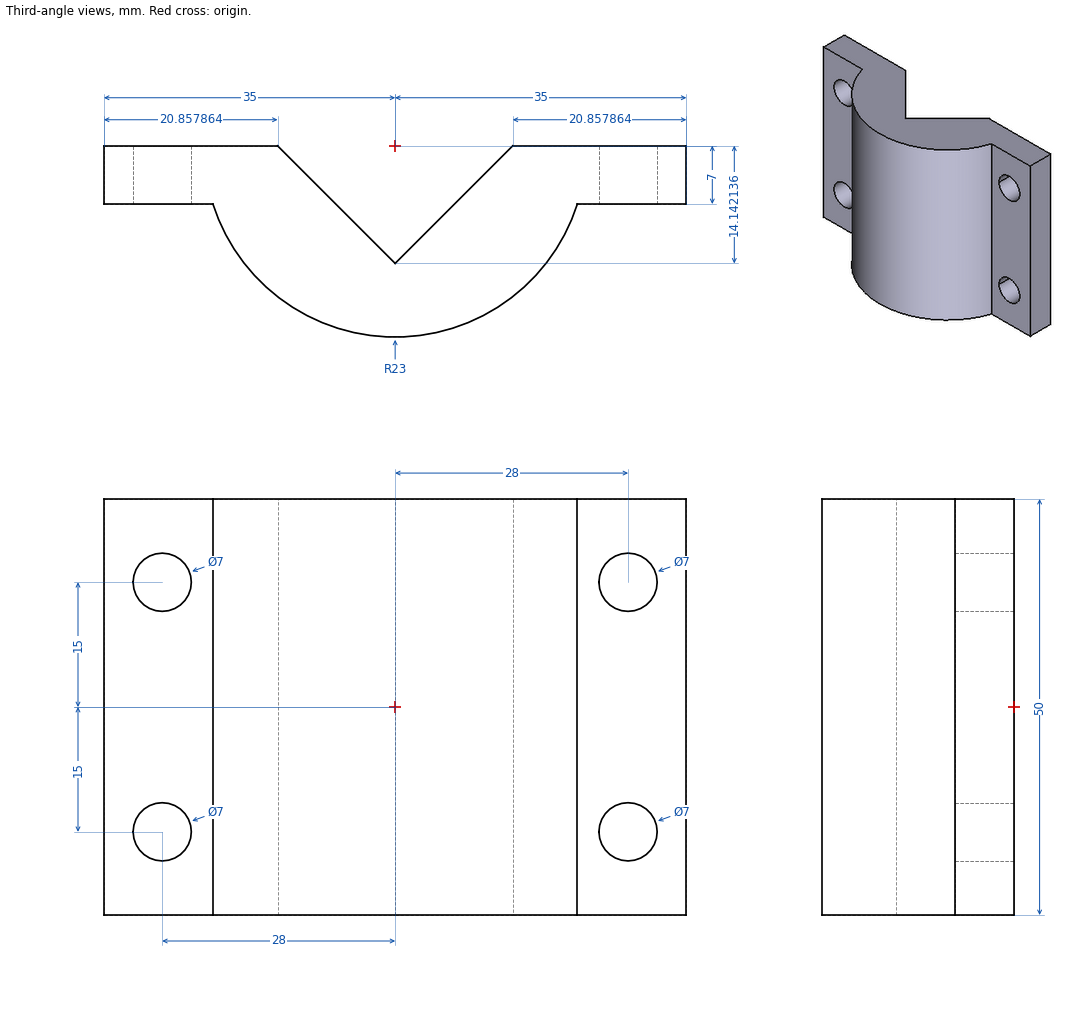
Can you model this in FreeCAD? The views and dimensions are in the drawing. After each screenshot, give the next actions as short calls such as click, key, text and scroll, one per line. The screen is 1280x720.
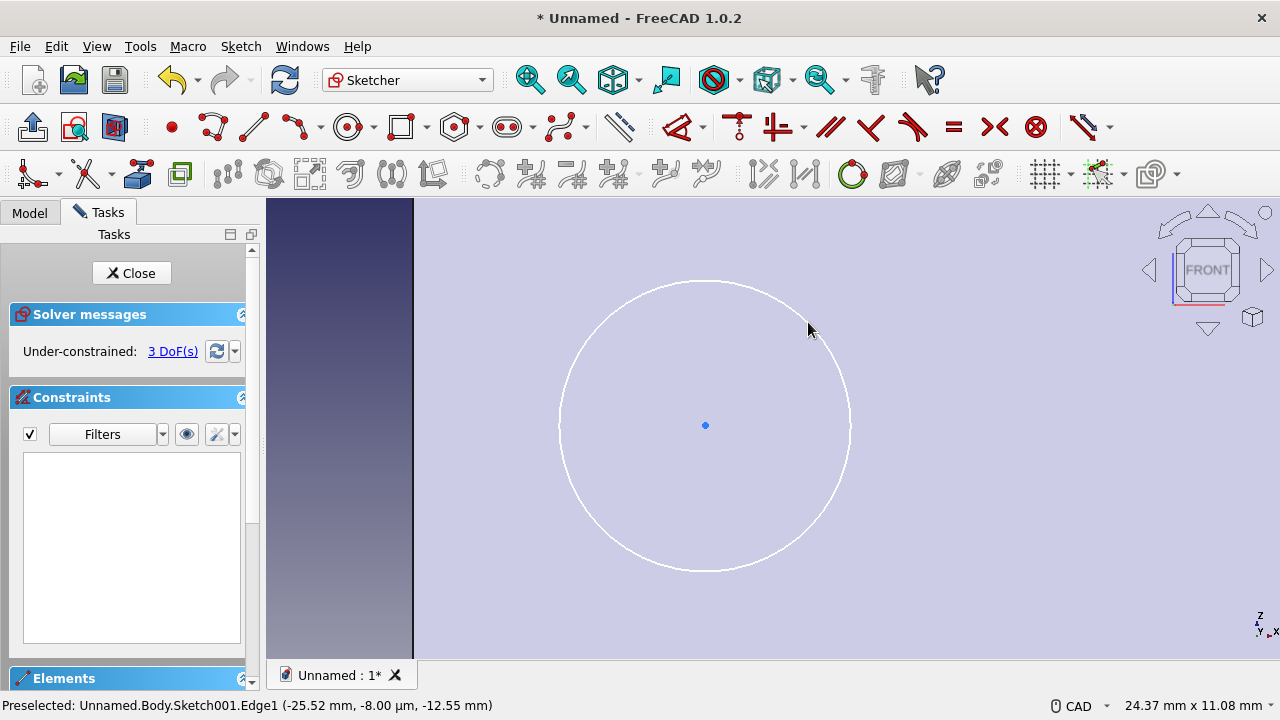
key(d)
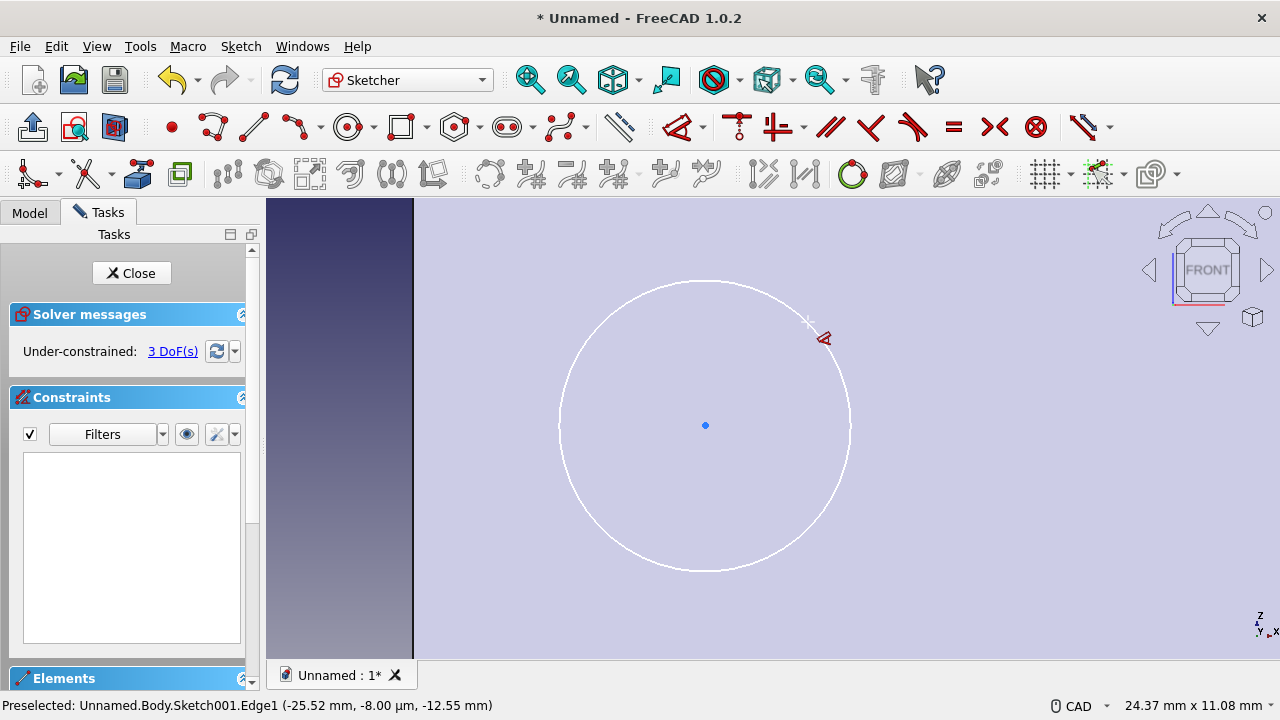
click(808, 323)
click(831, 300)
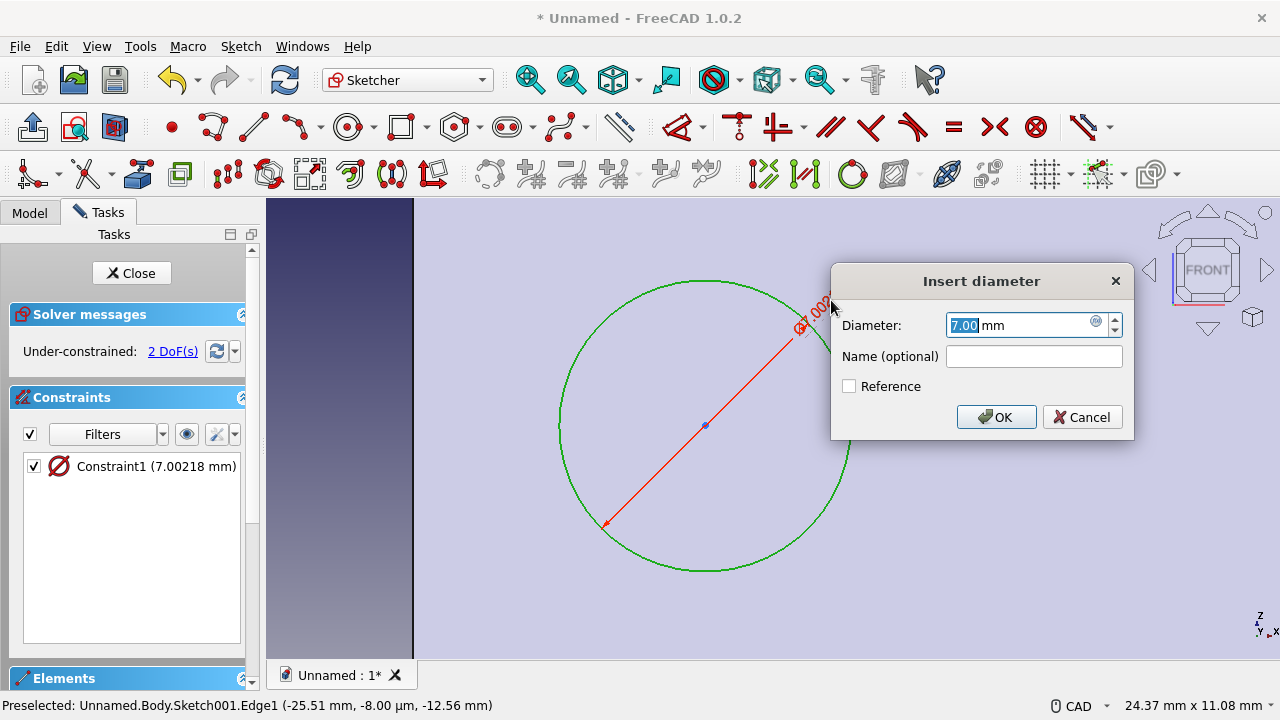
text(7)
key(Return)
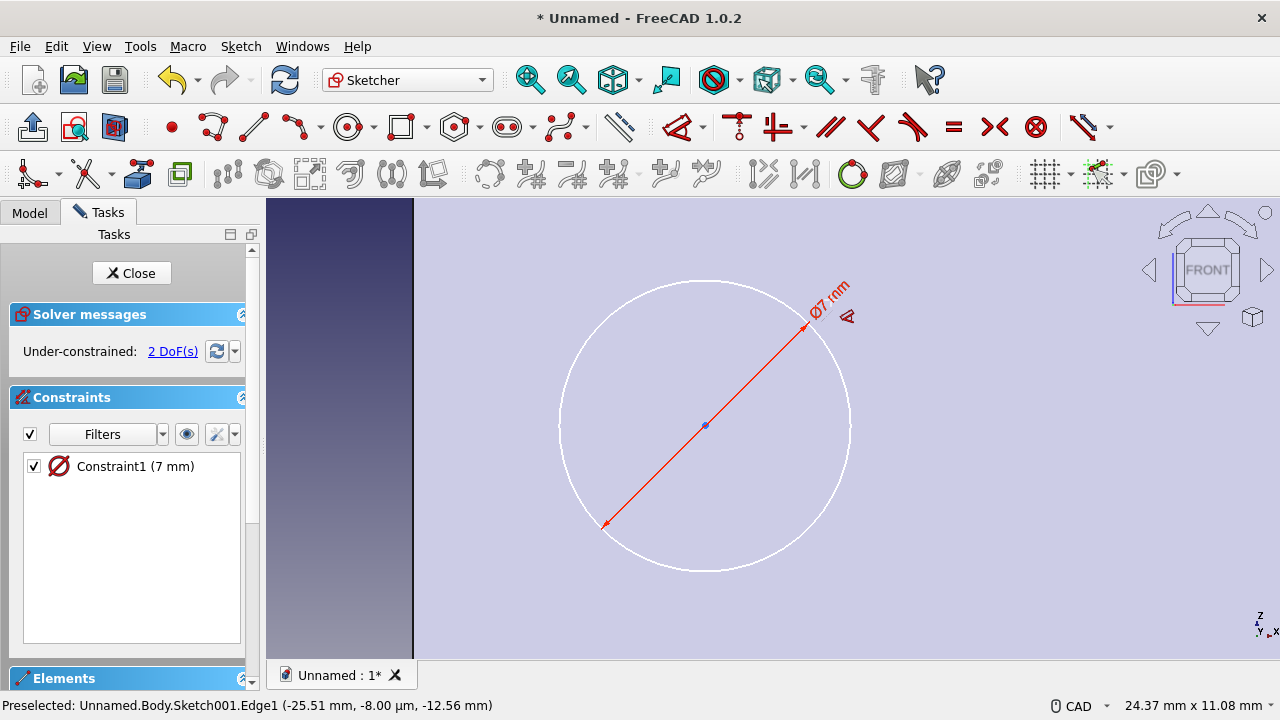
click(705, 426)
click(910, 460)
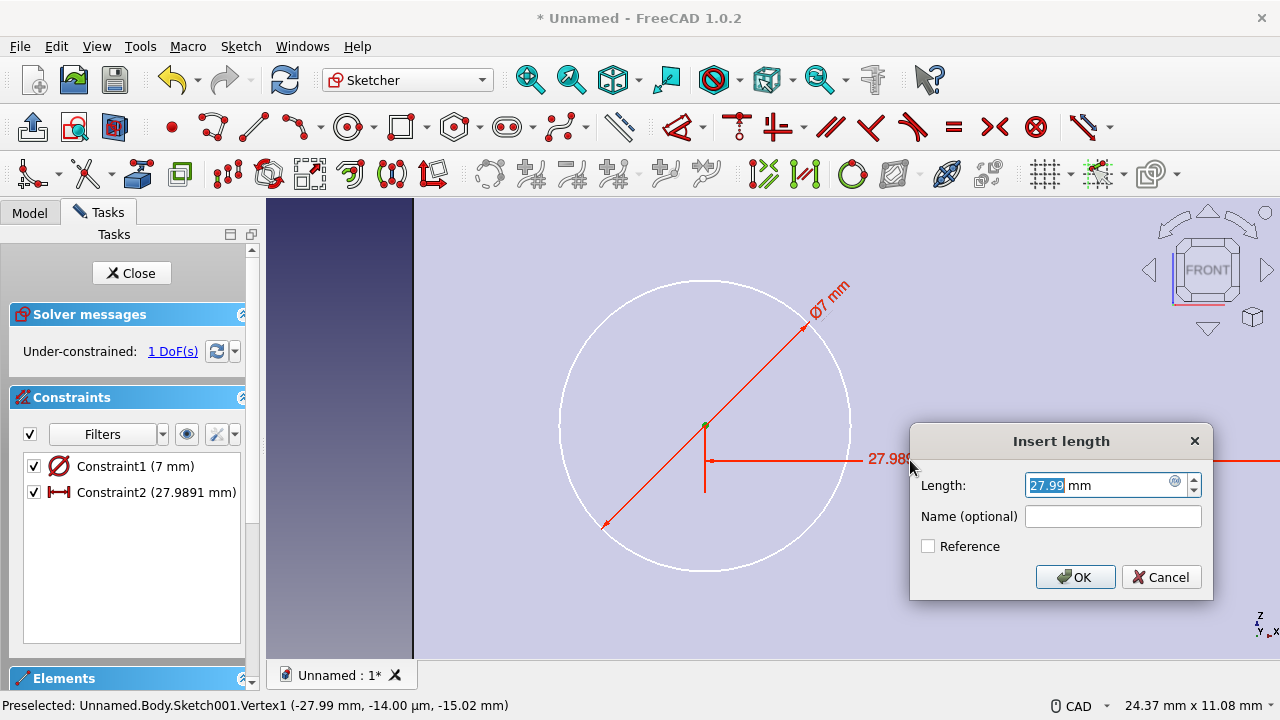
text(28)
key(Return)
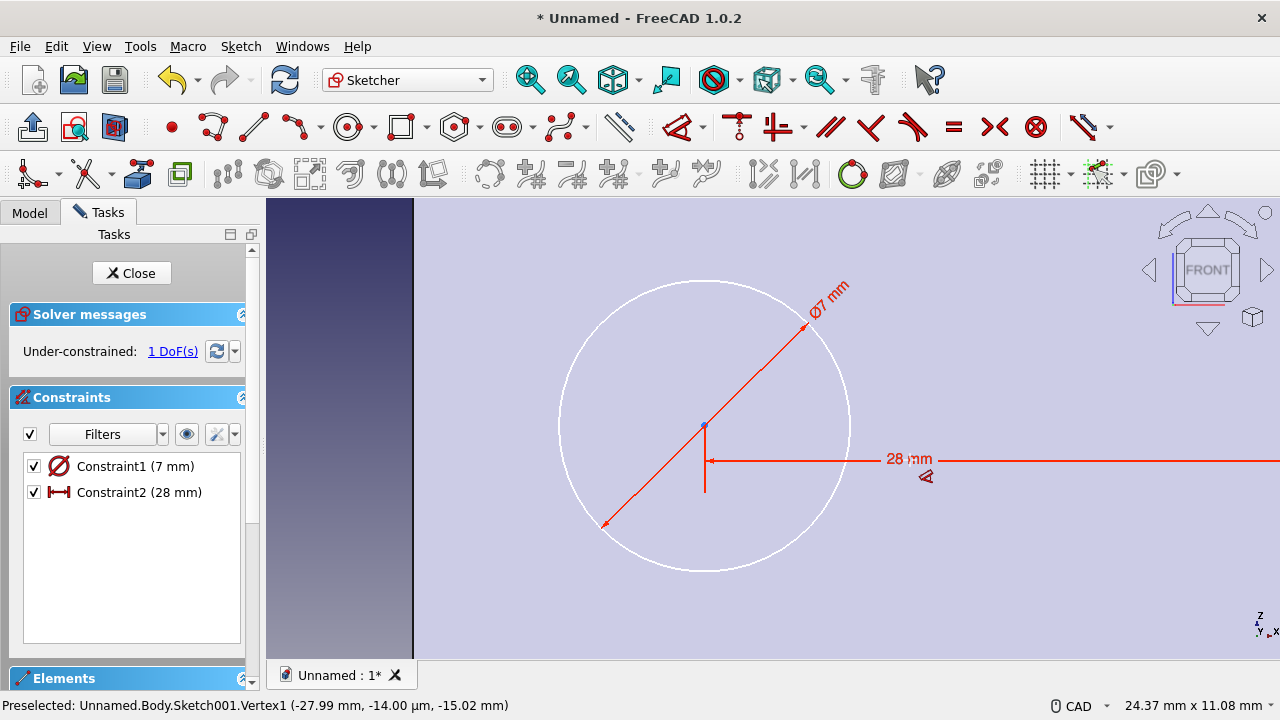
click(705, 426)
click(671, 326)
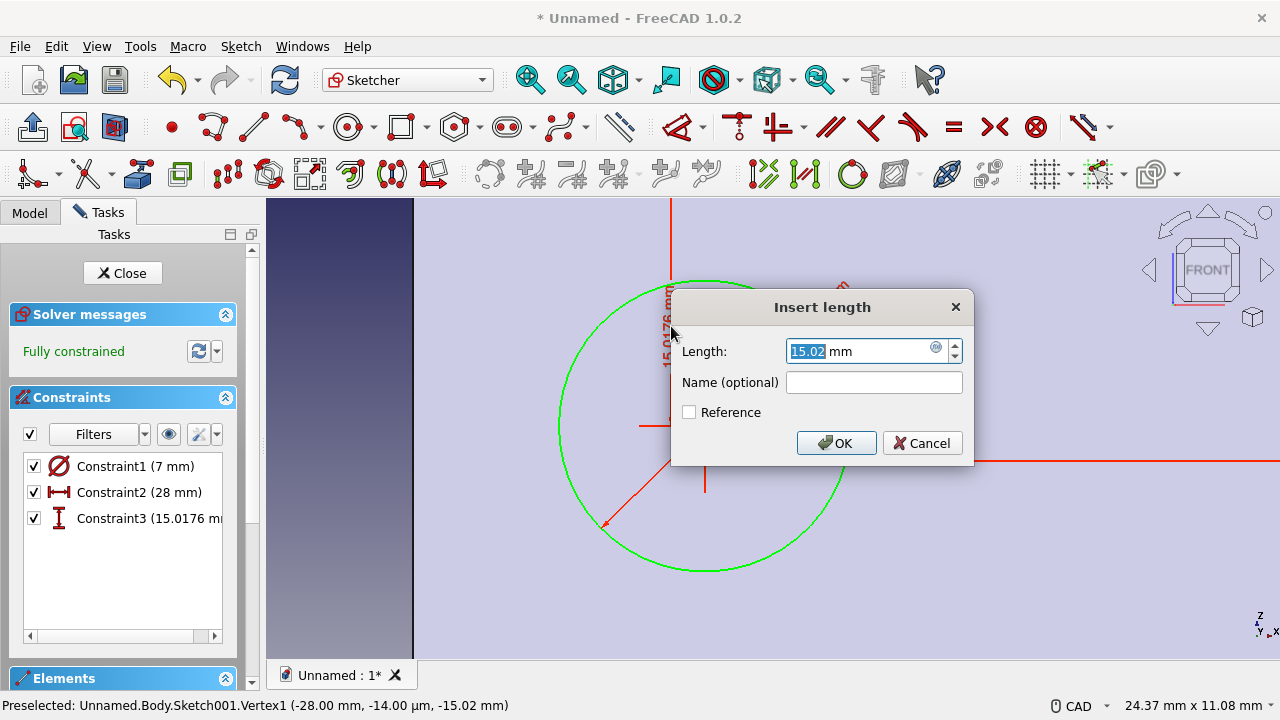
text(15)
key(Return)
key(Escape)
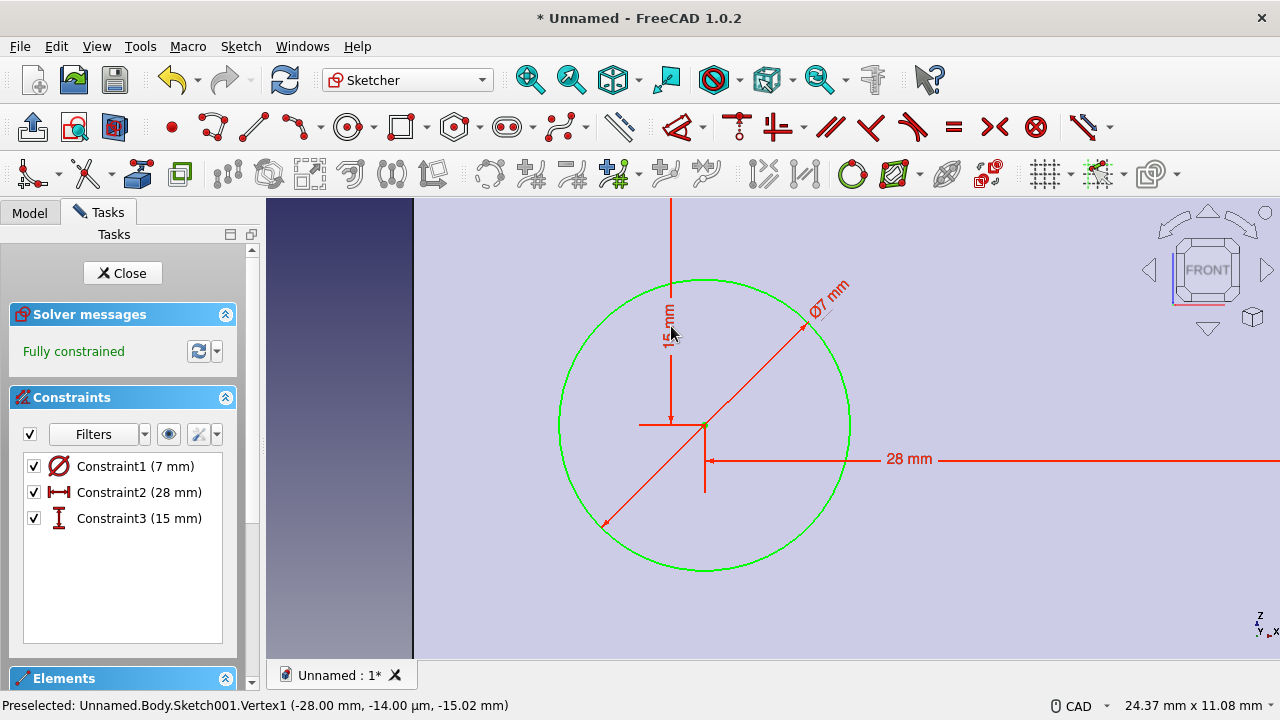
click(123, 273)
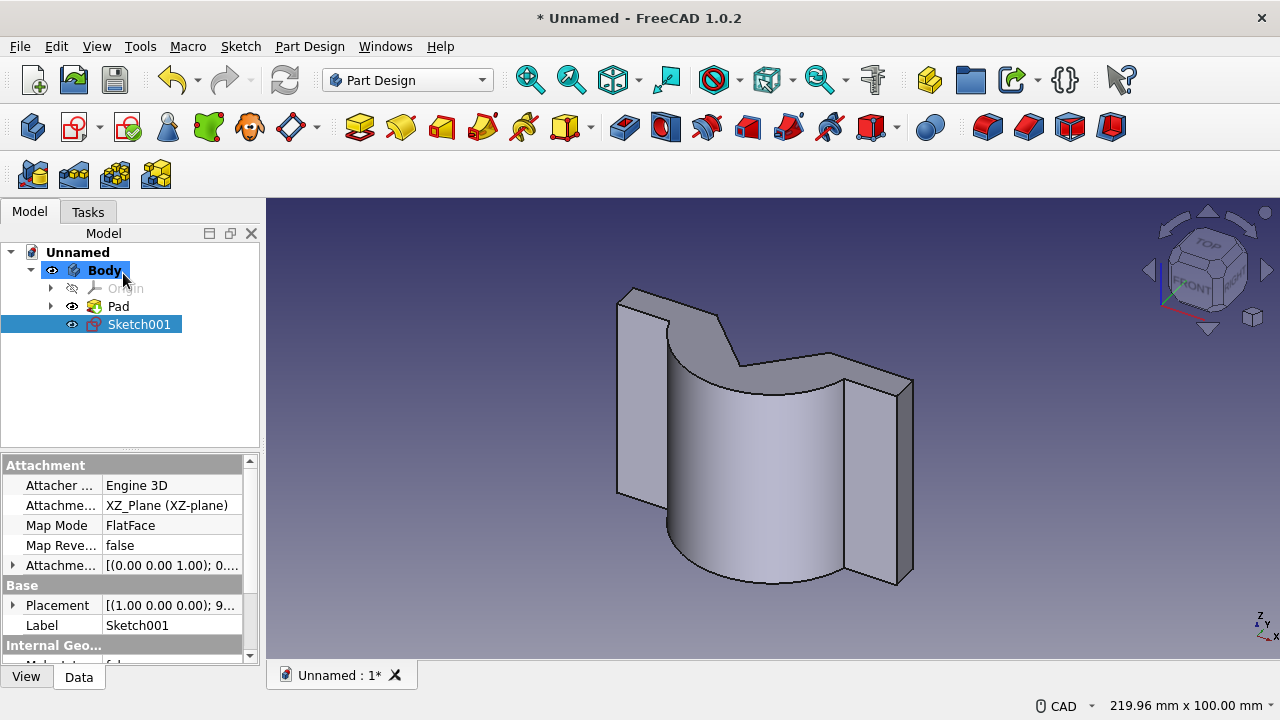
click(625, 128)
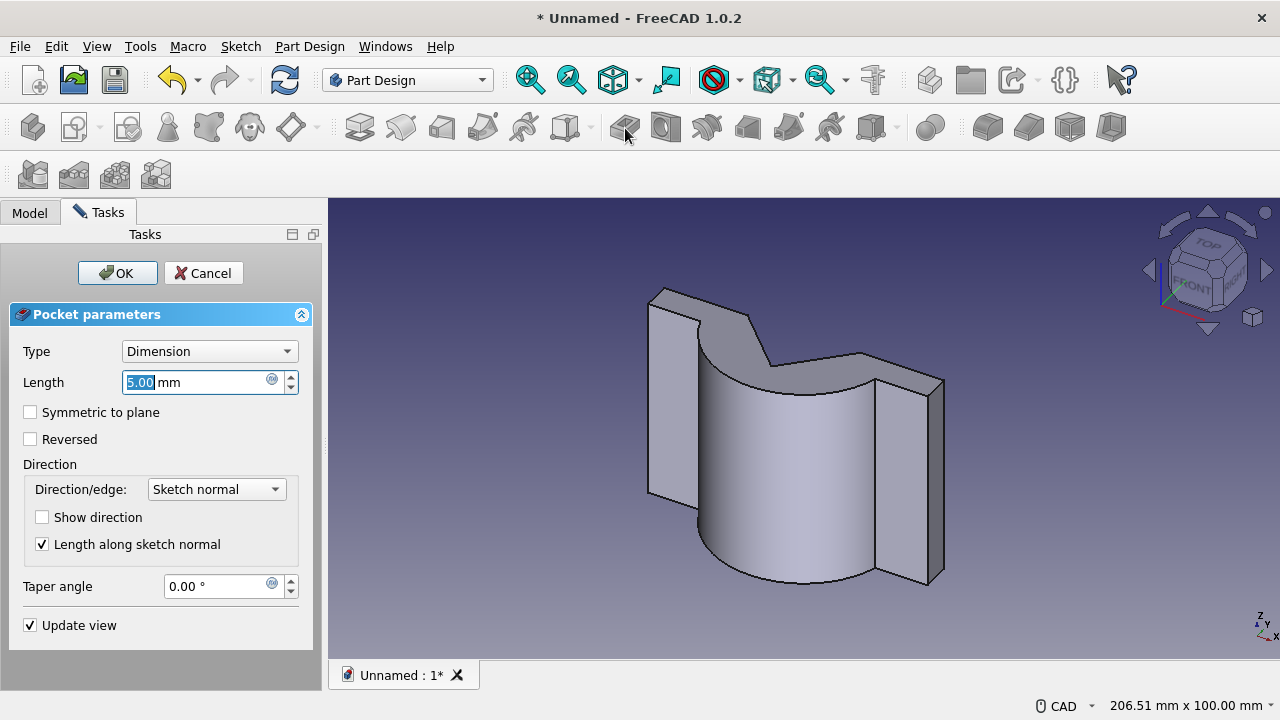
click(210, 352)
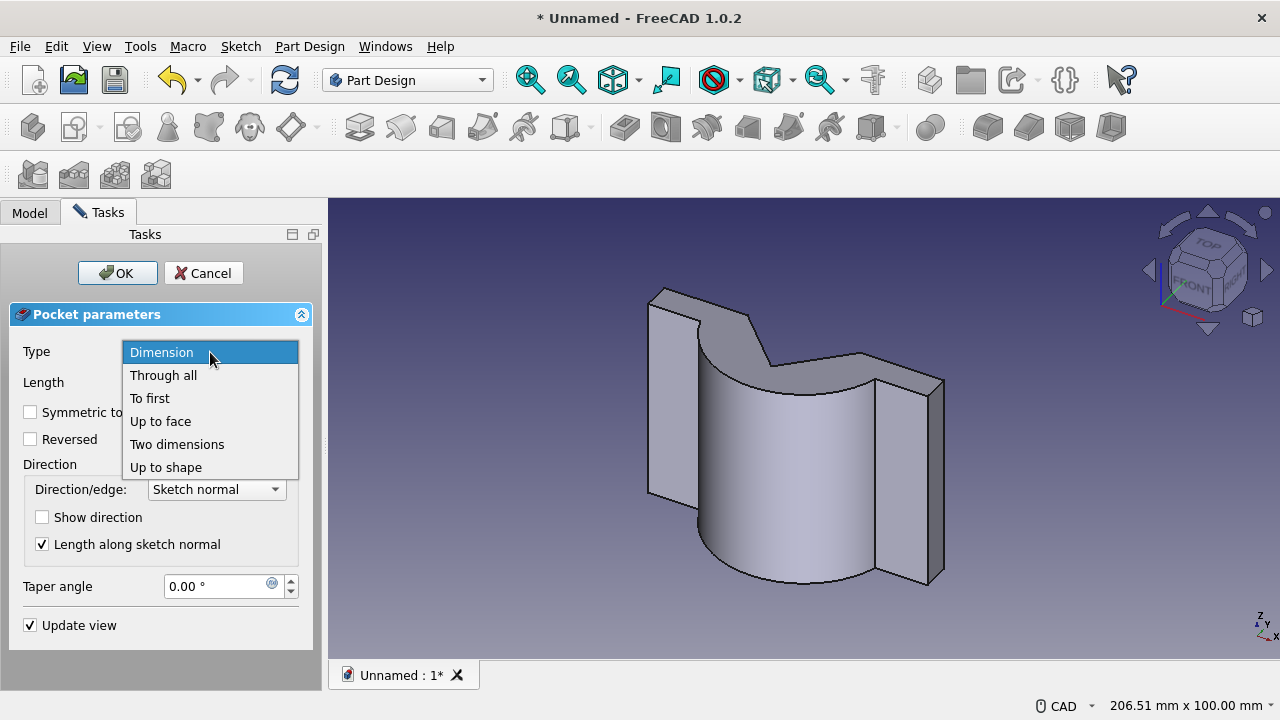
click(208, 398)